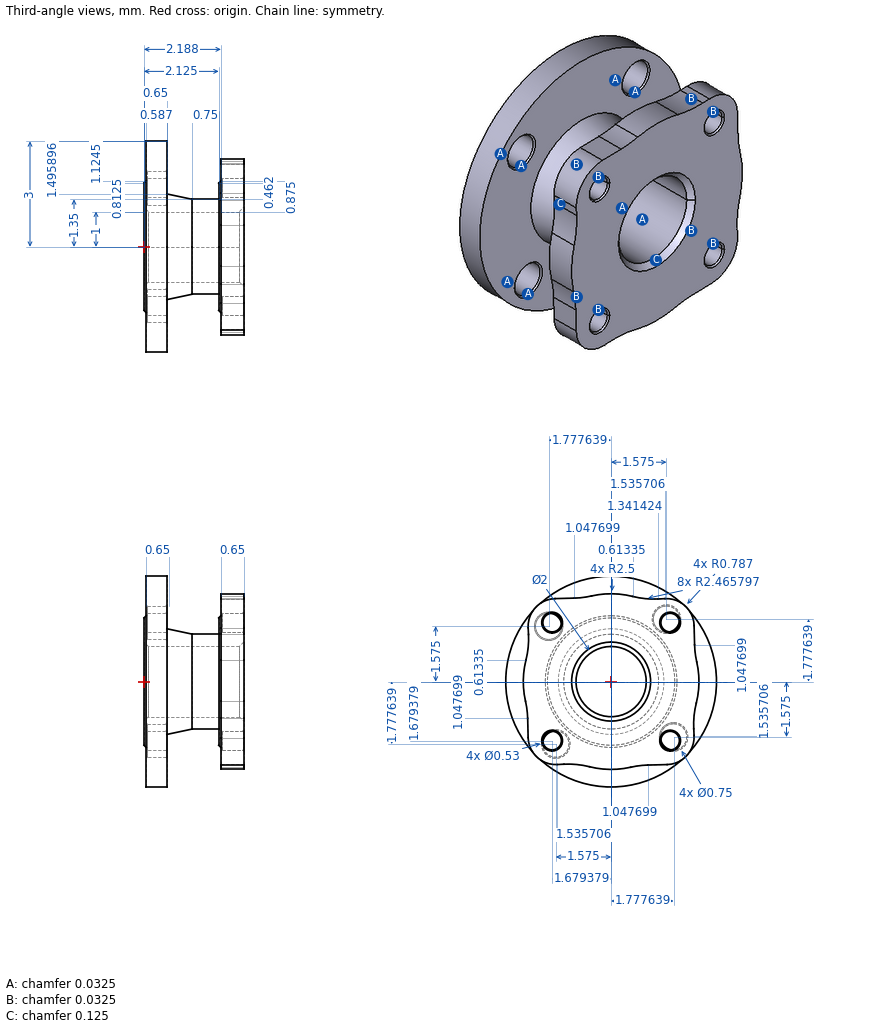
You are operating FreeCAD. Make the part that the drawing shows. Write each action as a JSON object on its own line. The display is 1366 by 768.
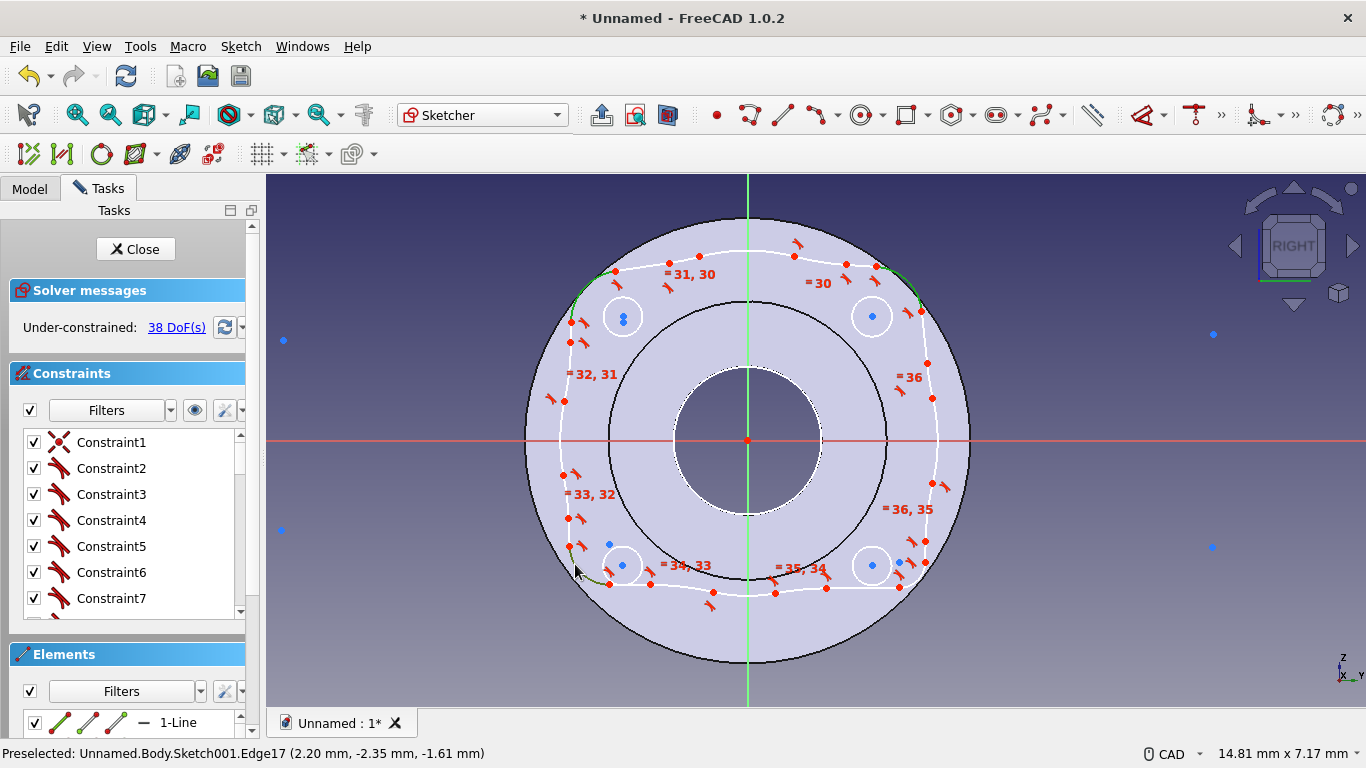
{"action": "left_click", "coordinate": [911, 585]}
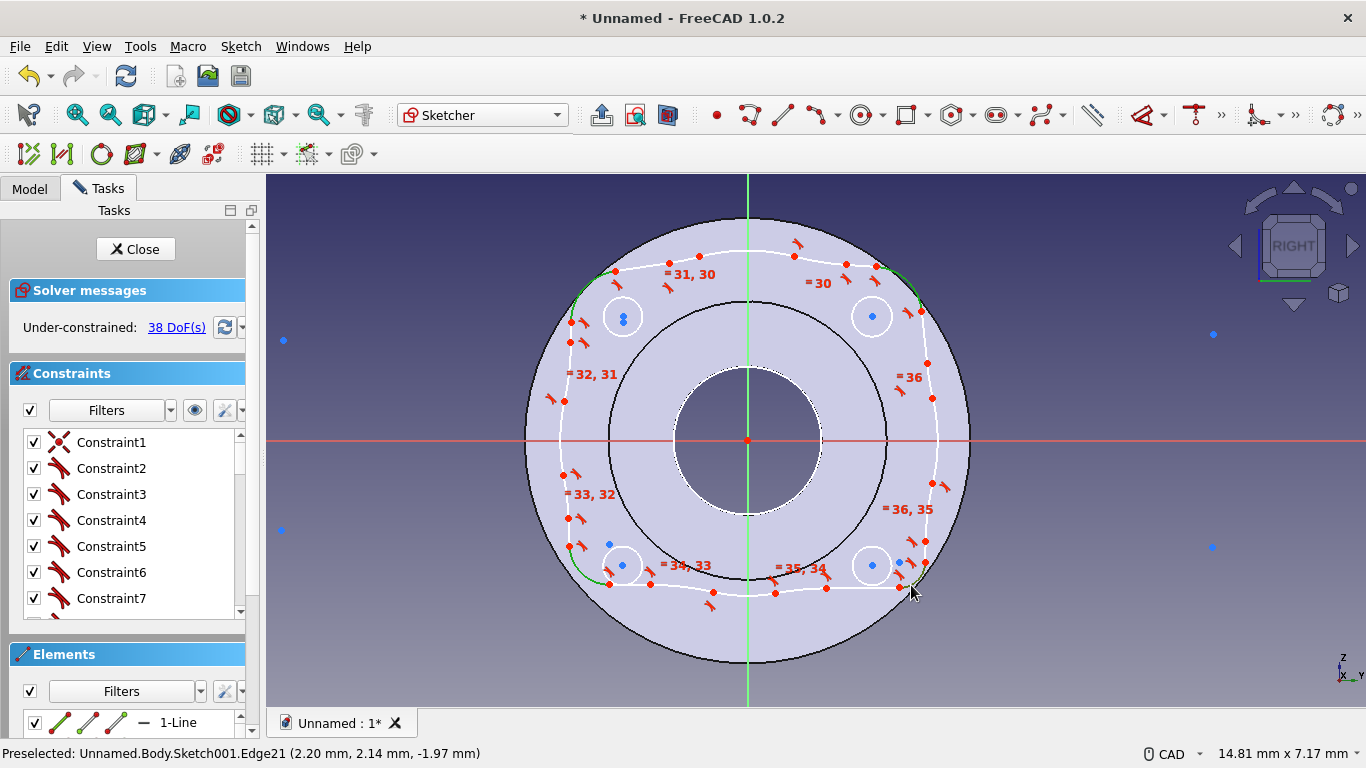
{"action": "key", "text": "e"}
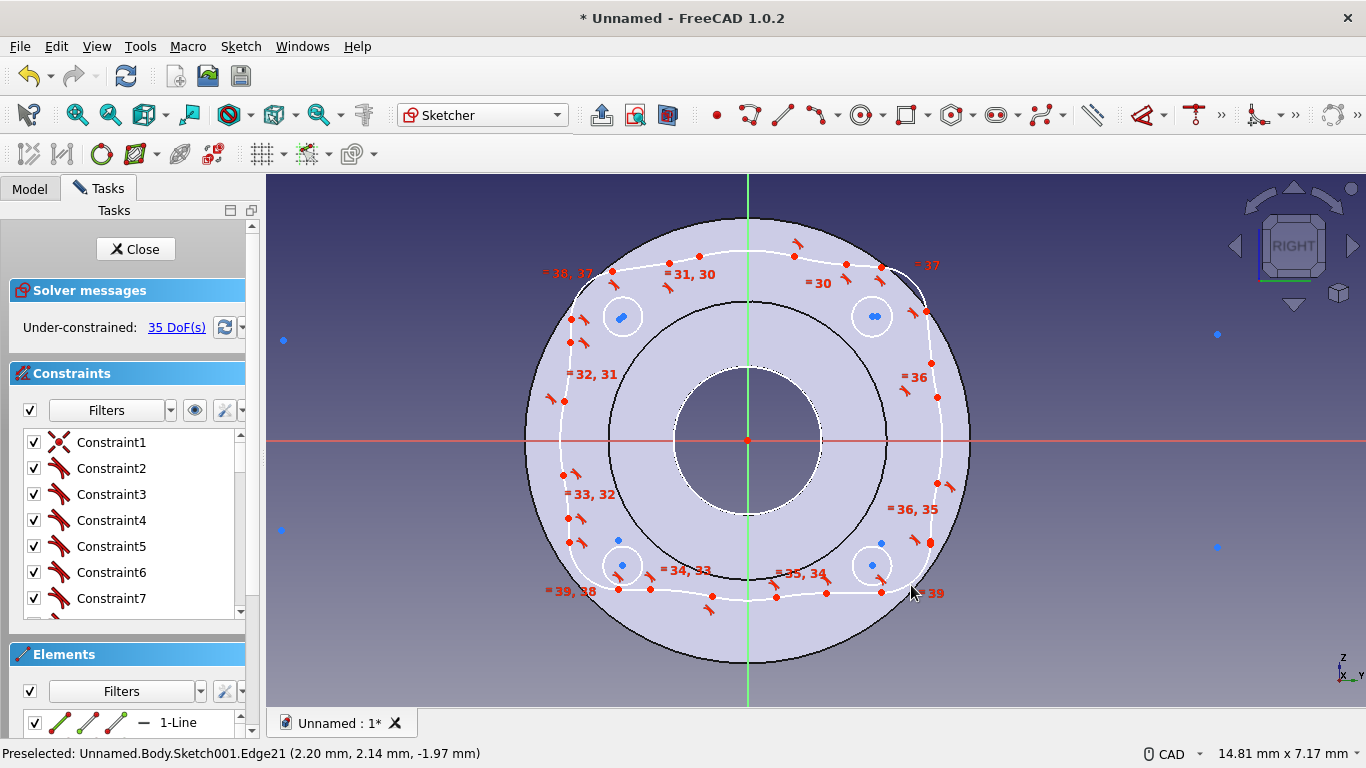
{"action": "left_click", "coordinate": [766, 252]}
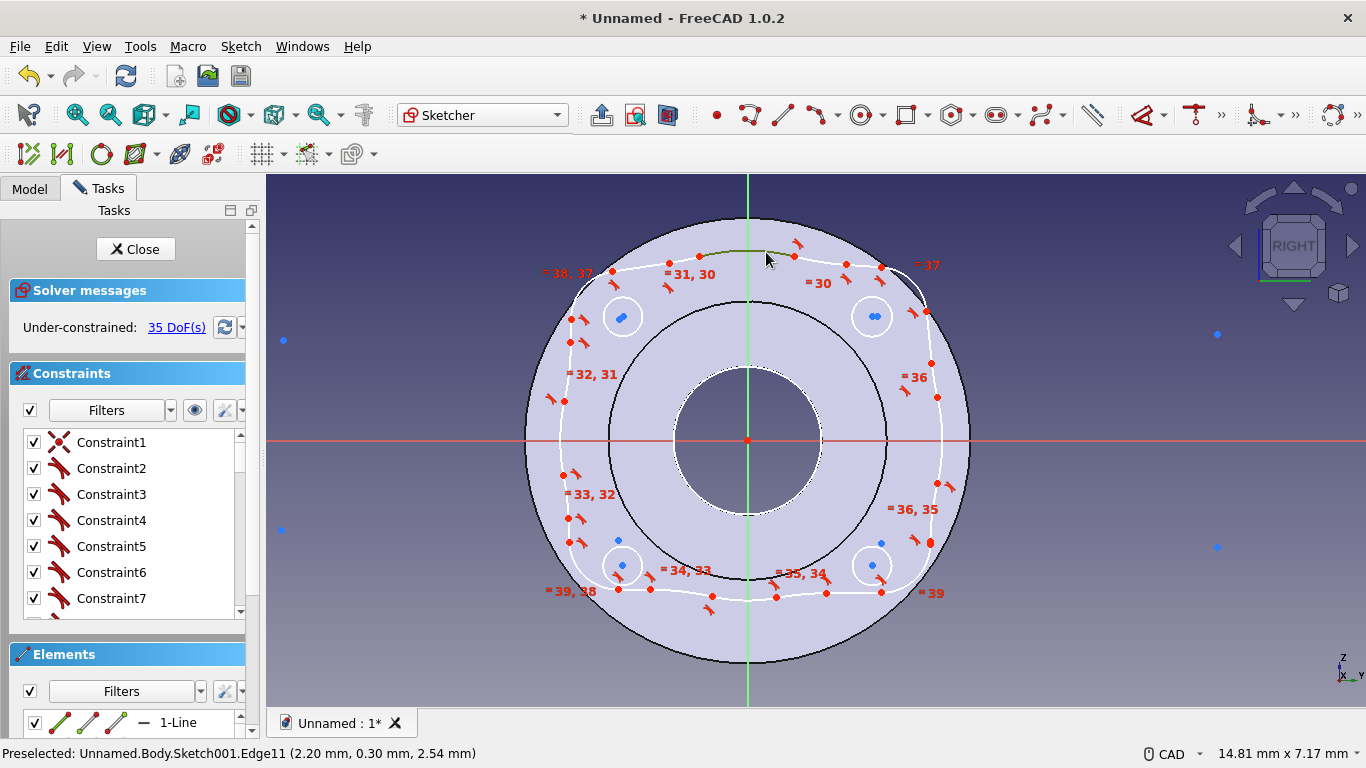
{"action": "left_click", "coordinate": [561, 424]}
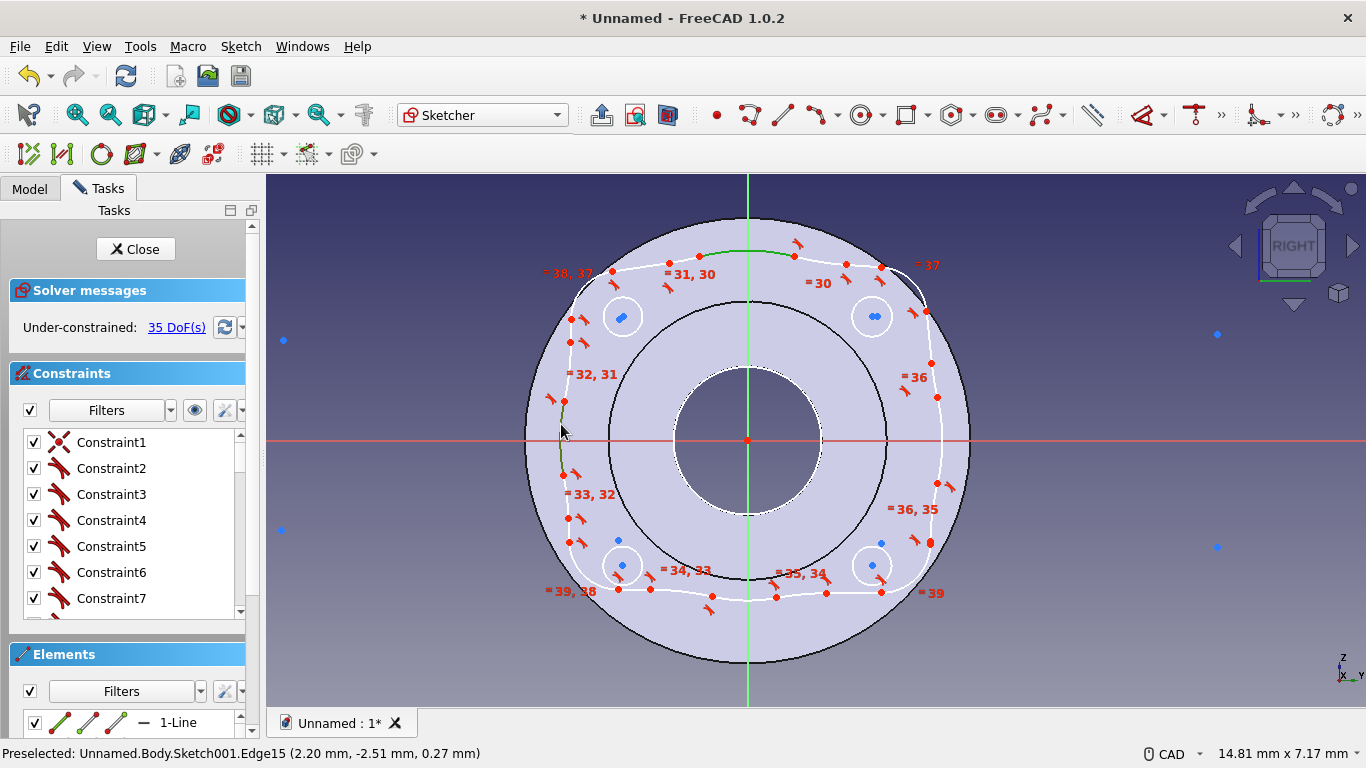
{"action": "left_click", "coordinate": [732, 600]}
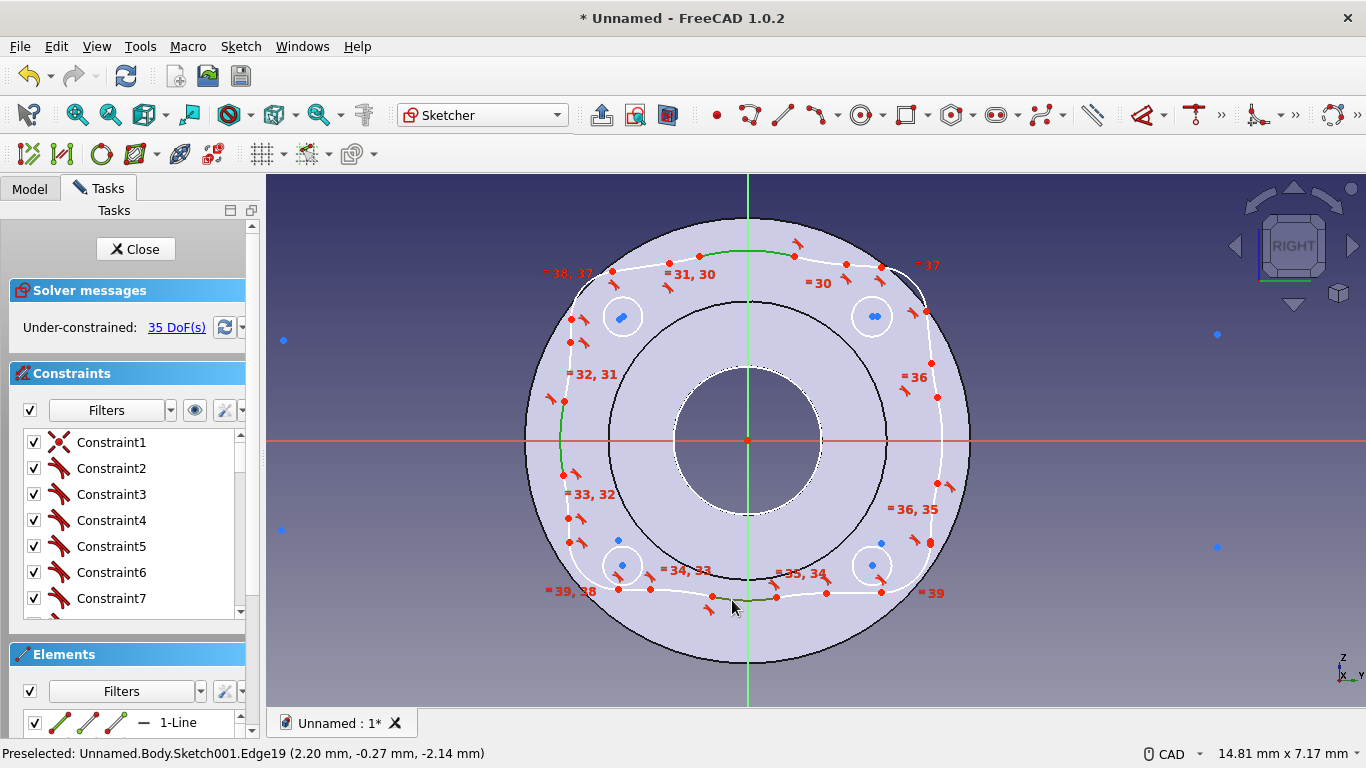
{"action": "left_click", "coordinate": [942, 458]}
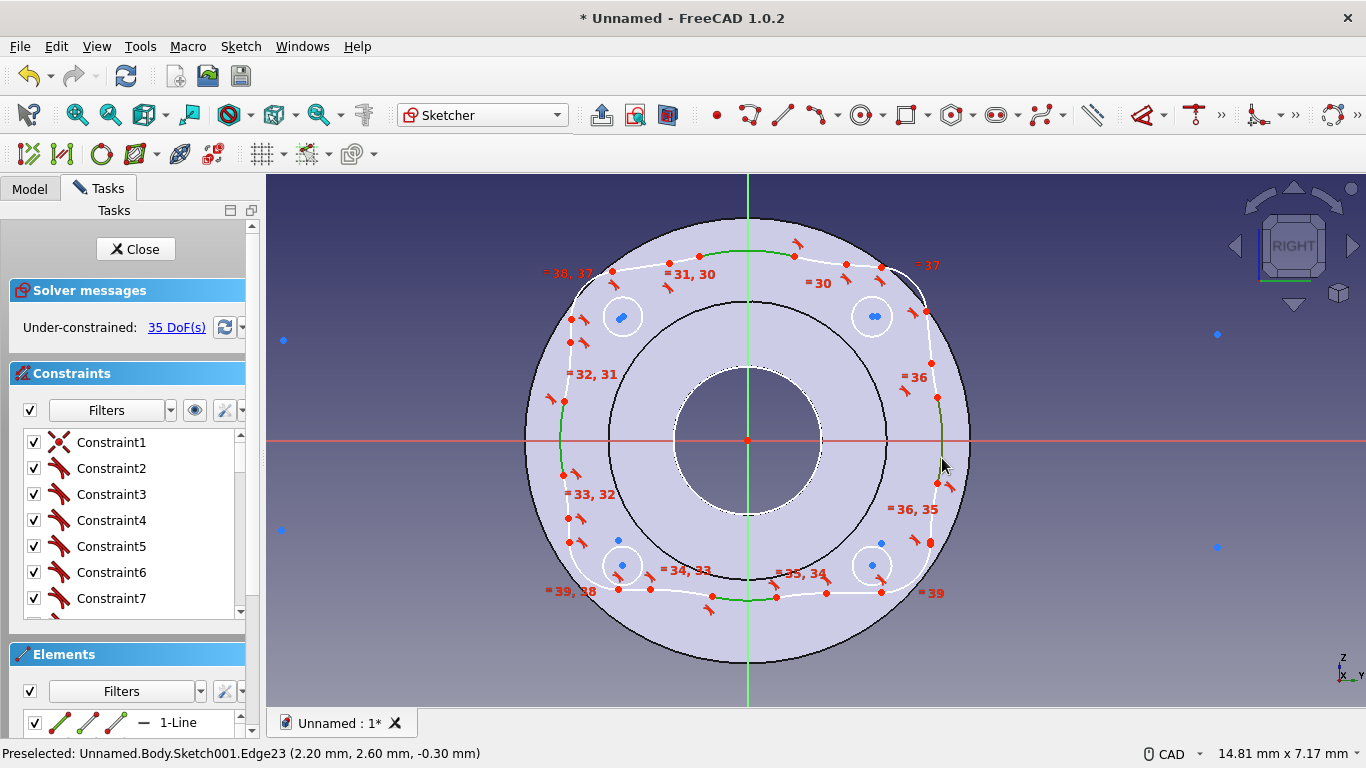
{"action": "key", "text": "e"}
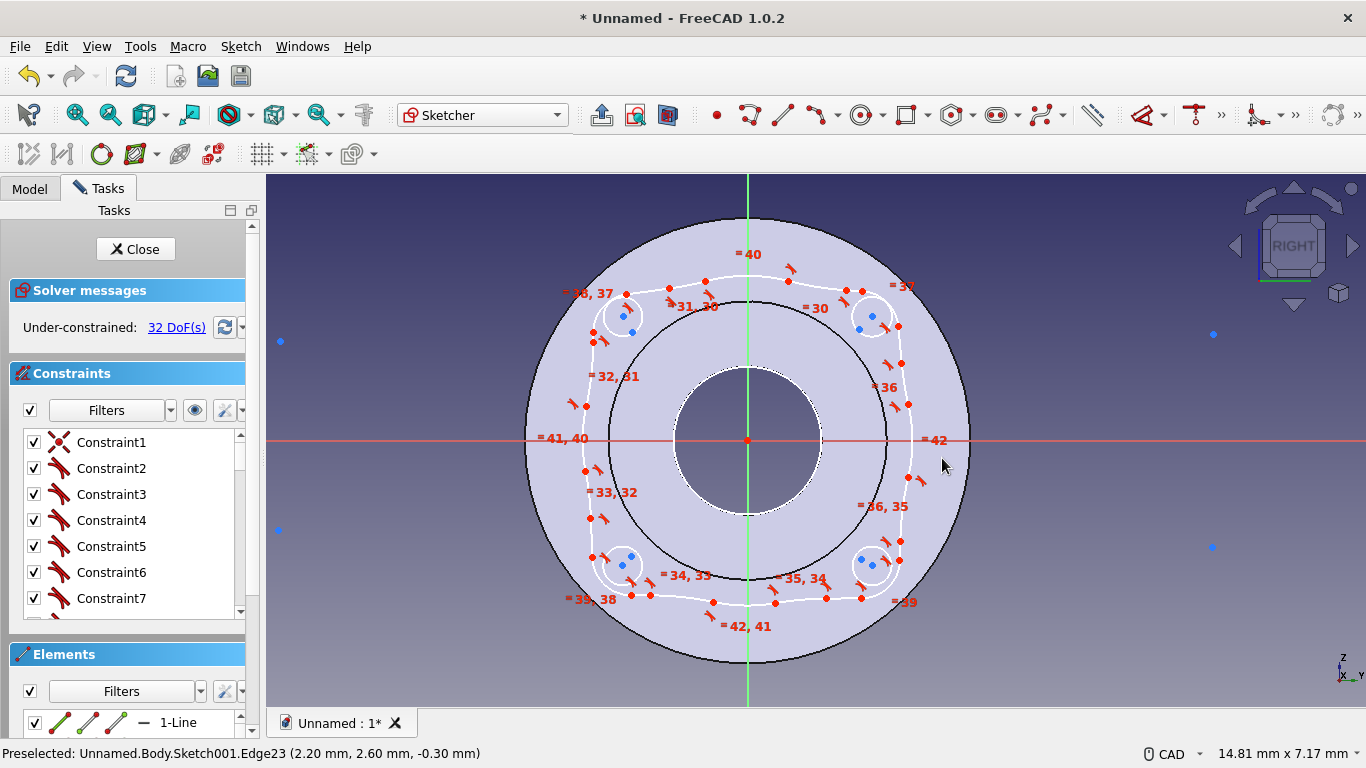
{"action": "left_click", "coordinate": [636, 552]}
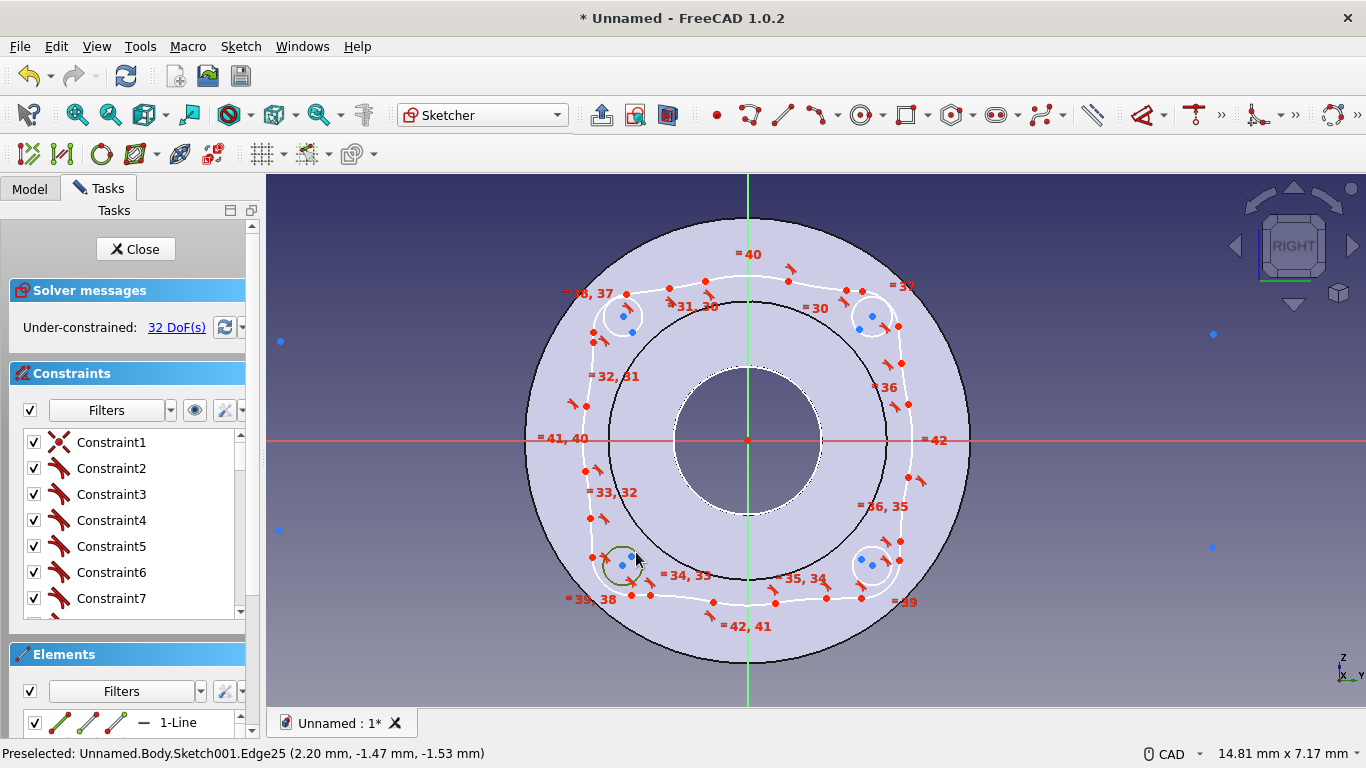
{"action": "scroll", "coordinate": [637, 303], "scroll_direction": "up", "scroll_amount": 2}